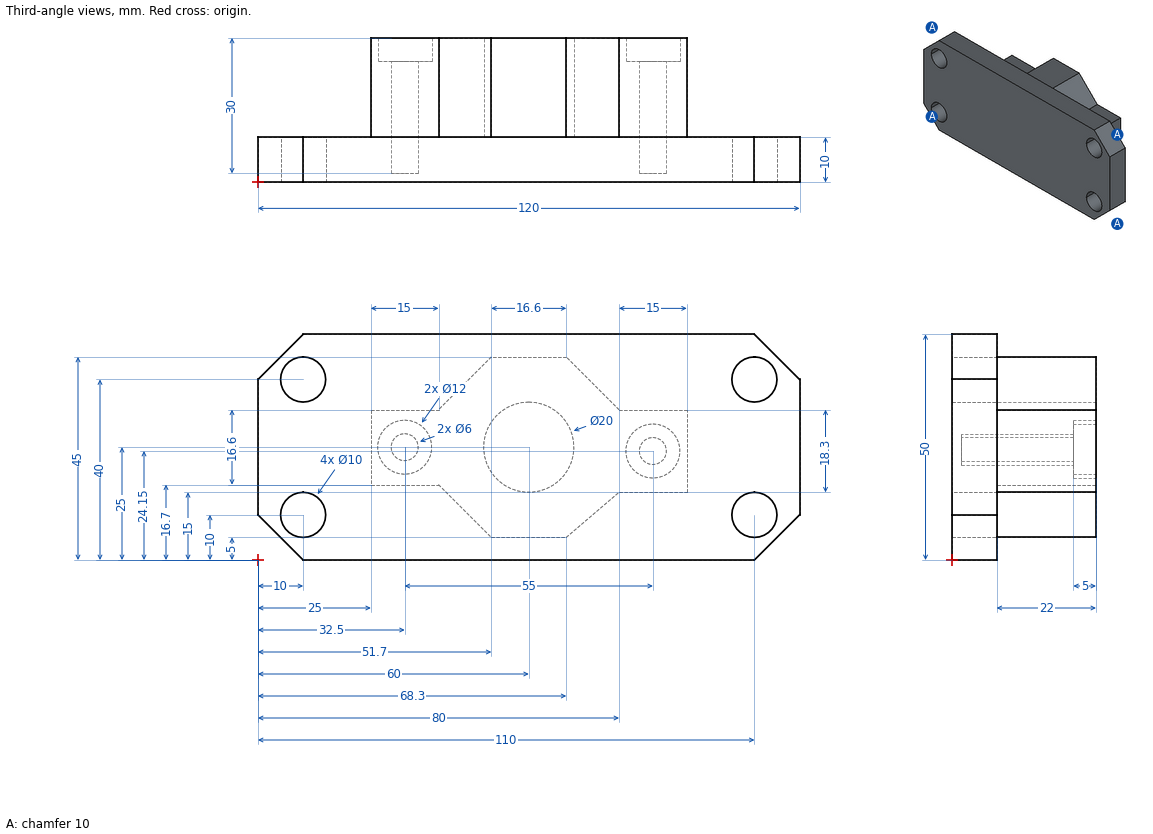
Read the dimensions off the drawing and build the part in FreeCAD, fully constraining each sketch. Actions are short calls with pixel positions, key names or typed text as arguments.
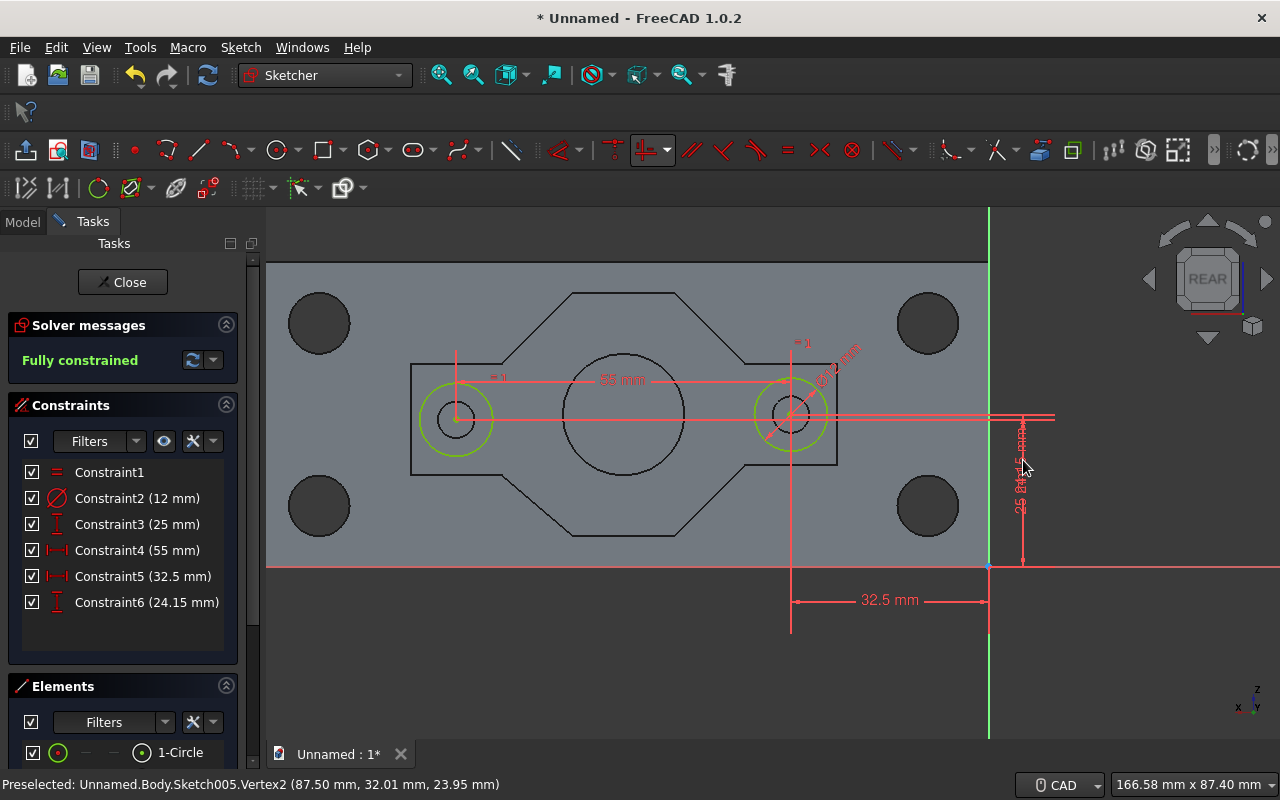
click(123, 282)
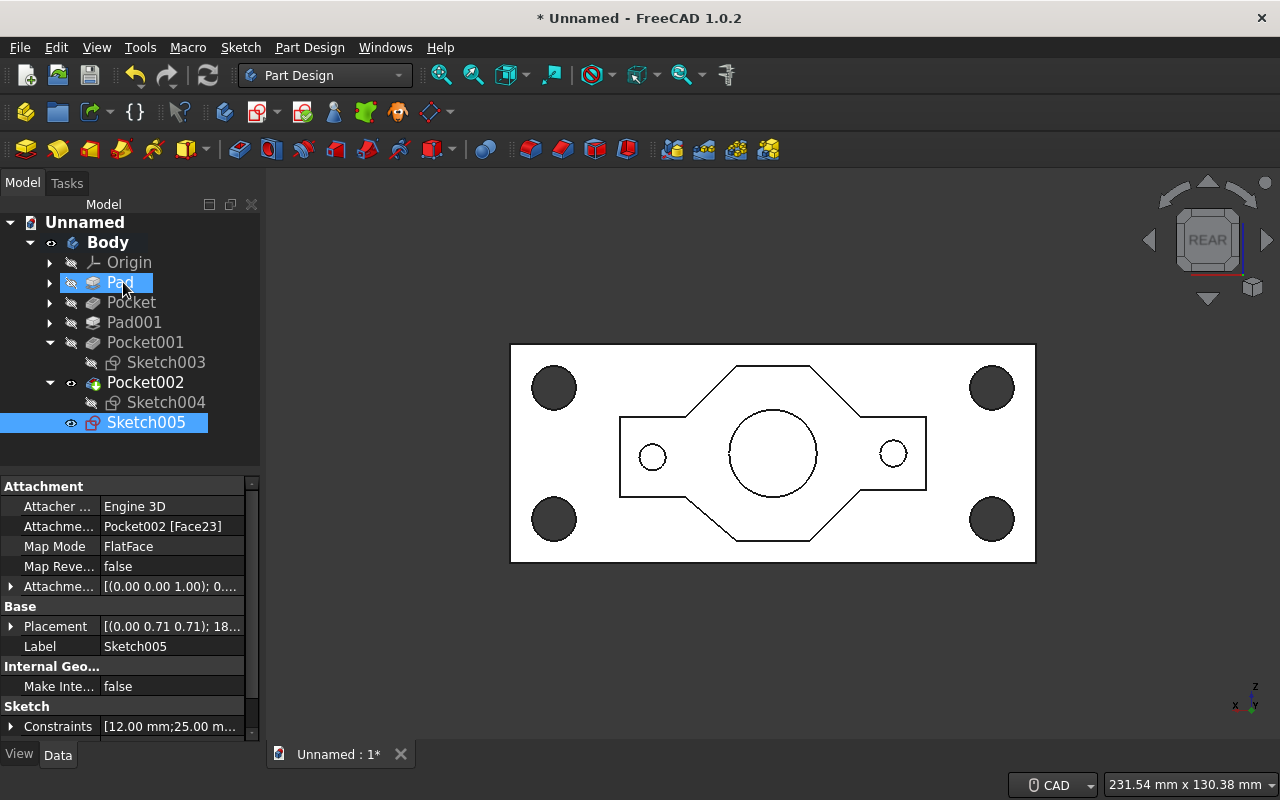
click(240, 150)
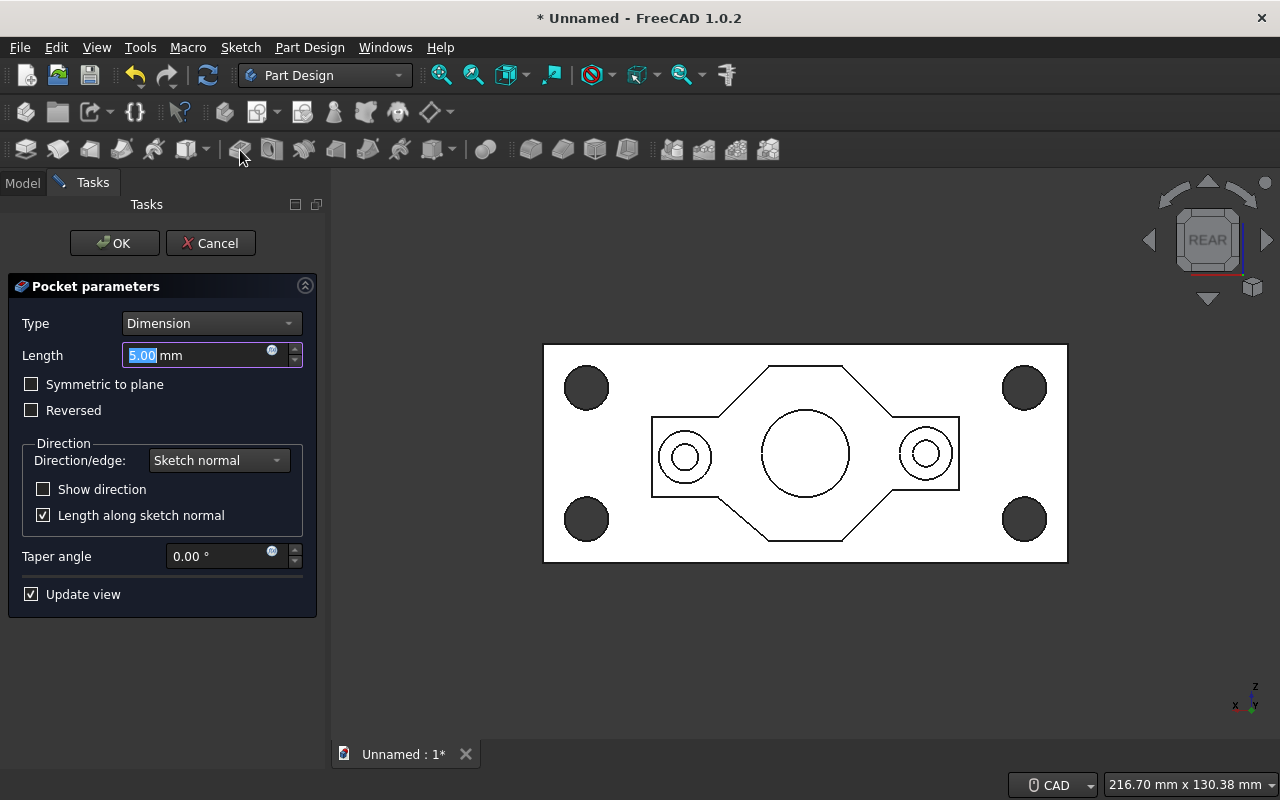
text(5)
key(Tab)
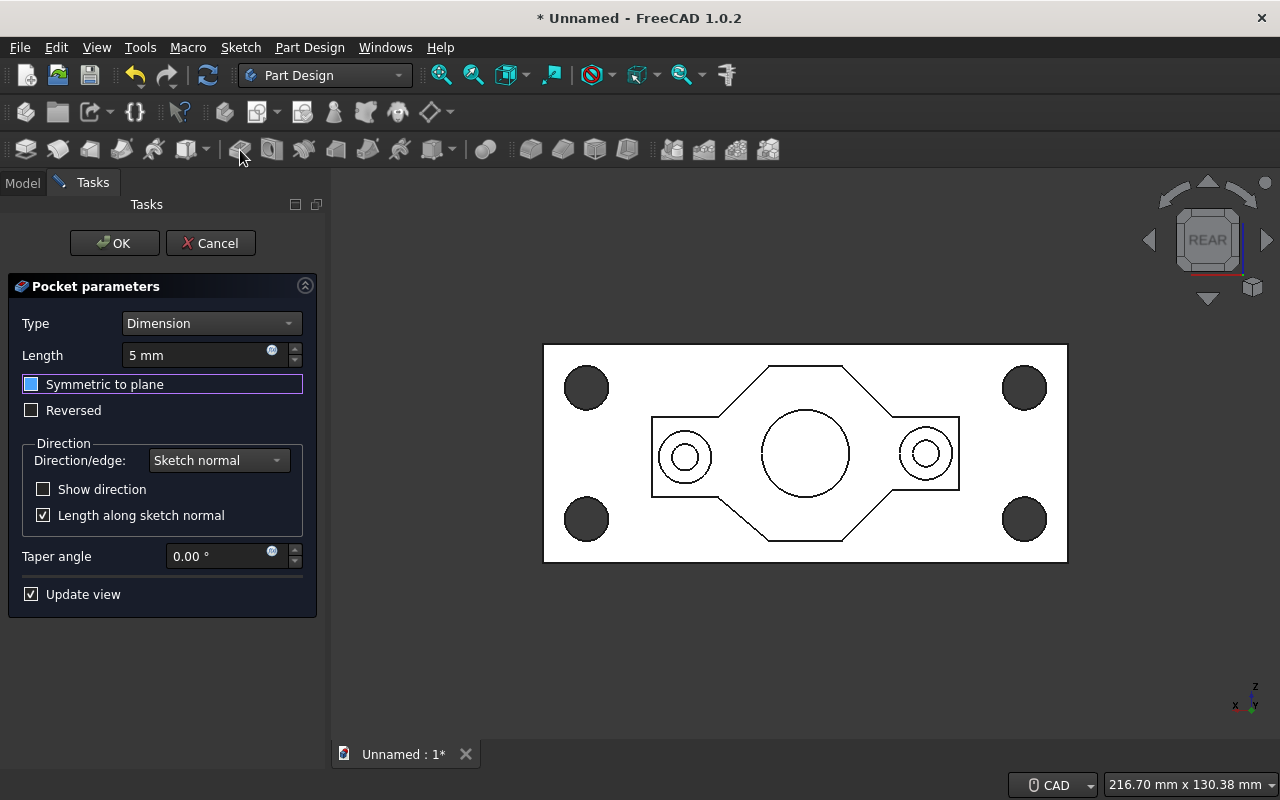
click(115, 243)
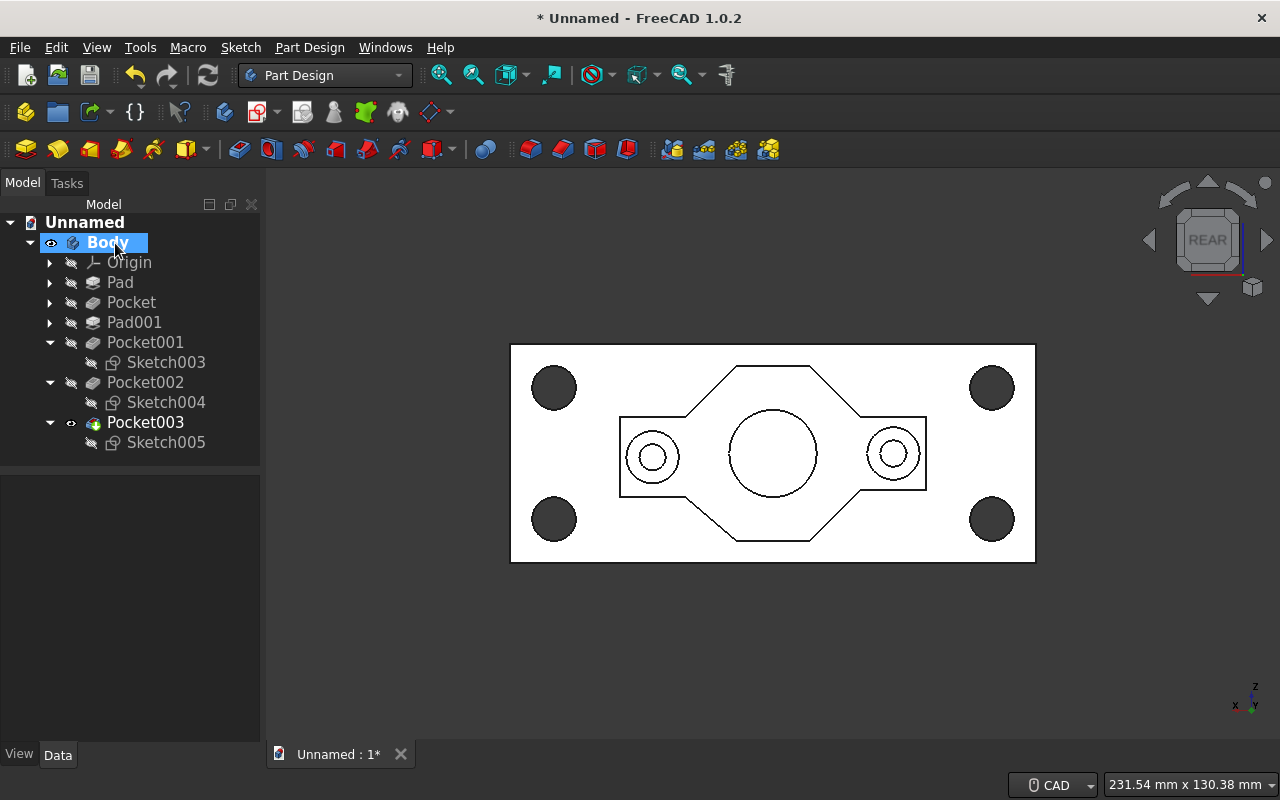
key(0)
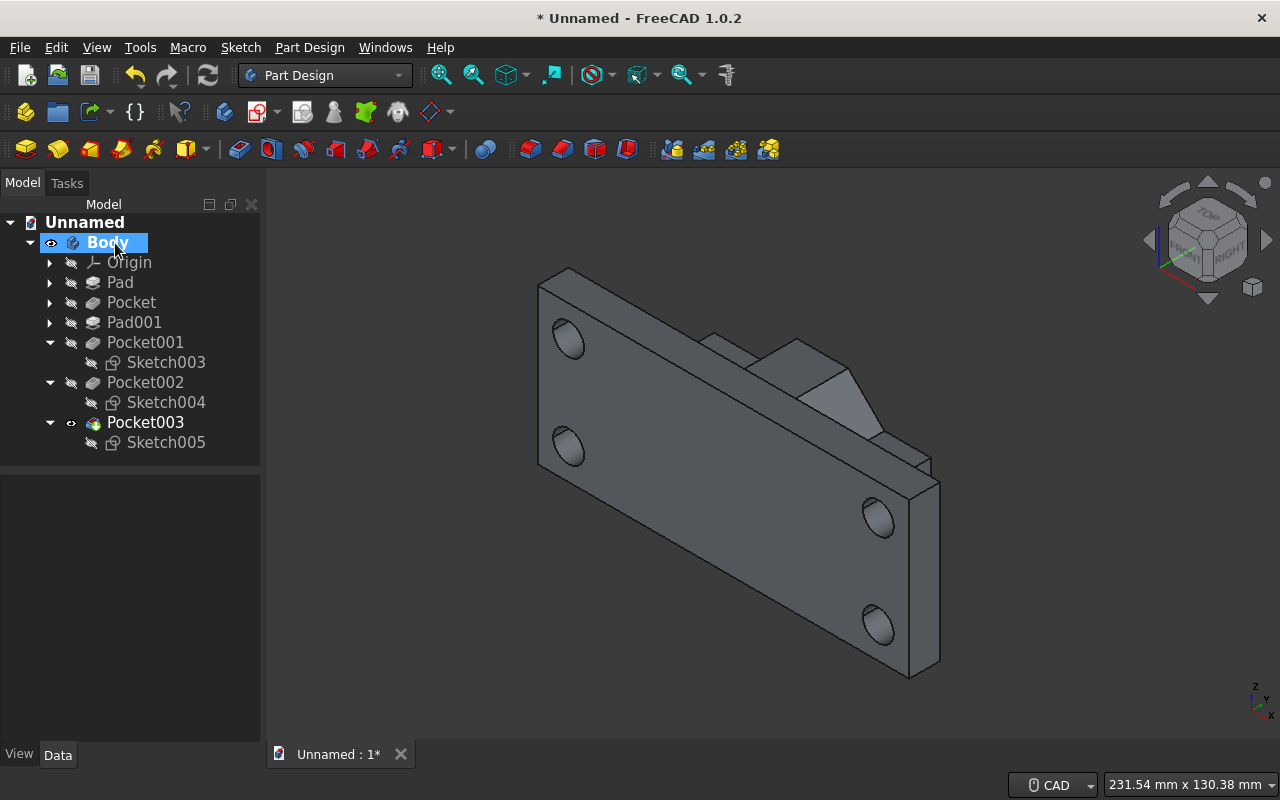
click(925, 490)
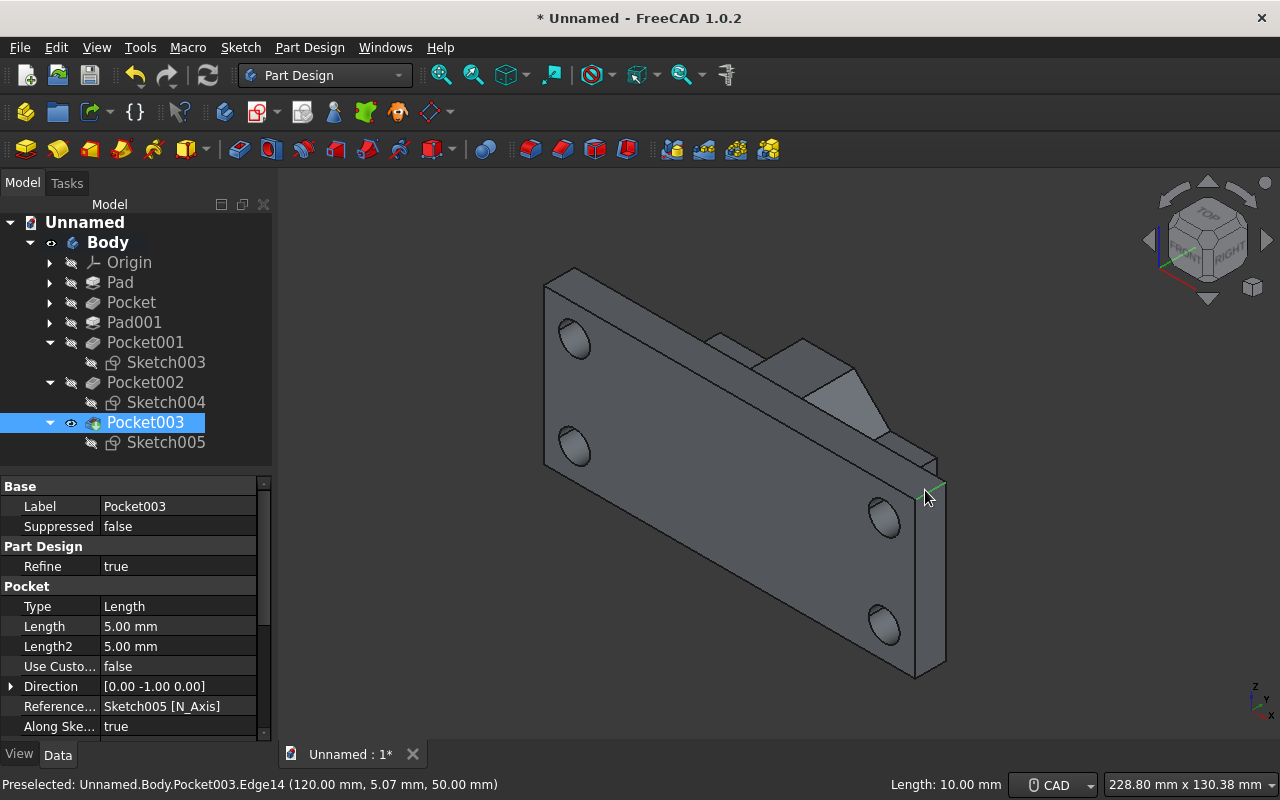
key(2)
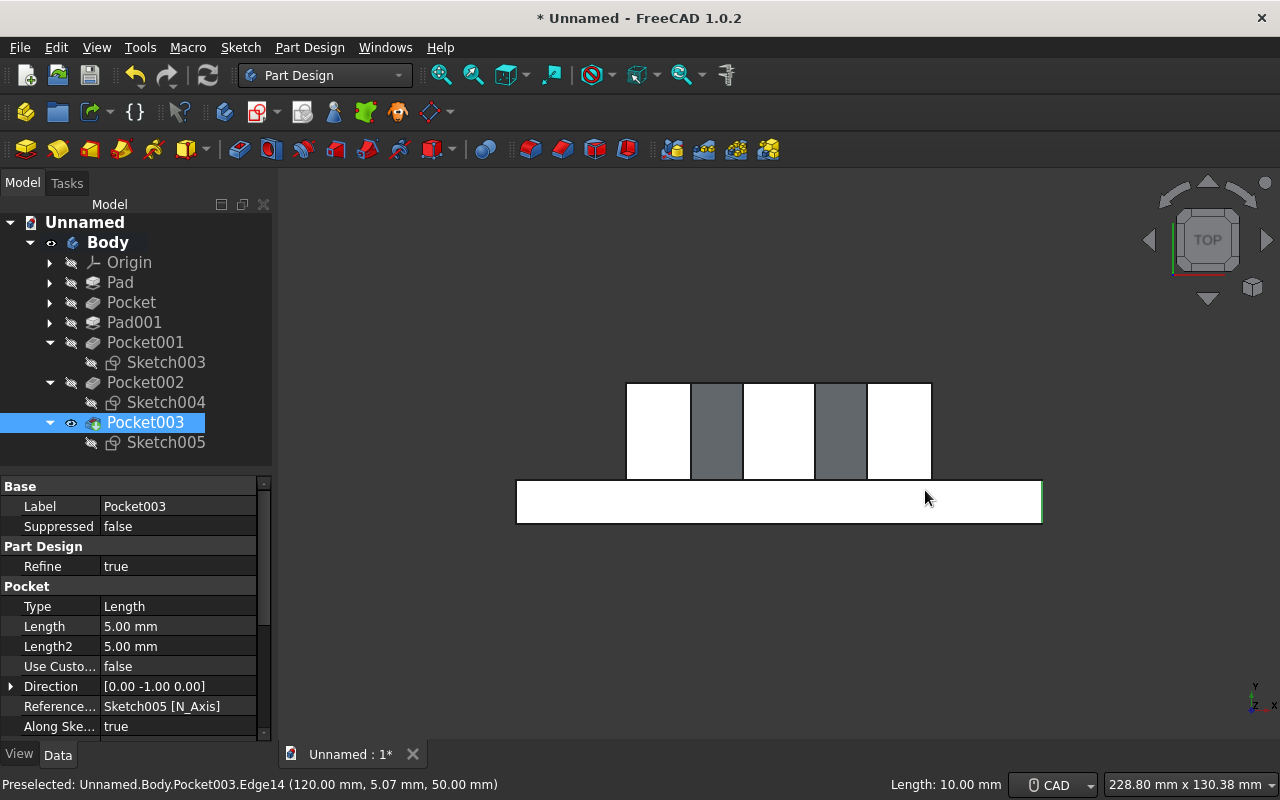
click(516, 501, ctrl)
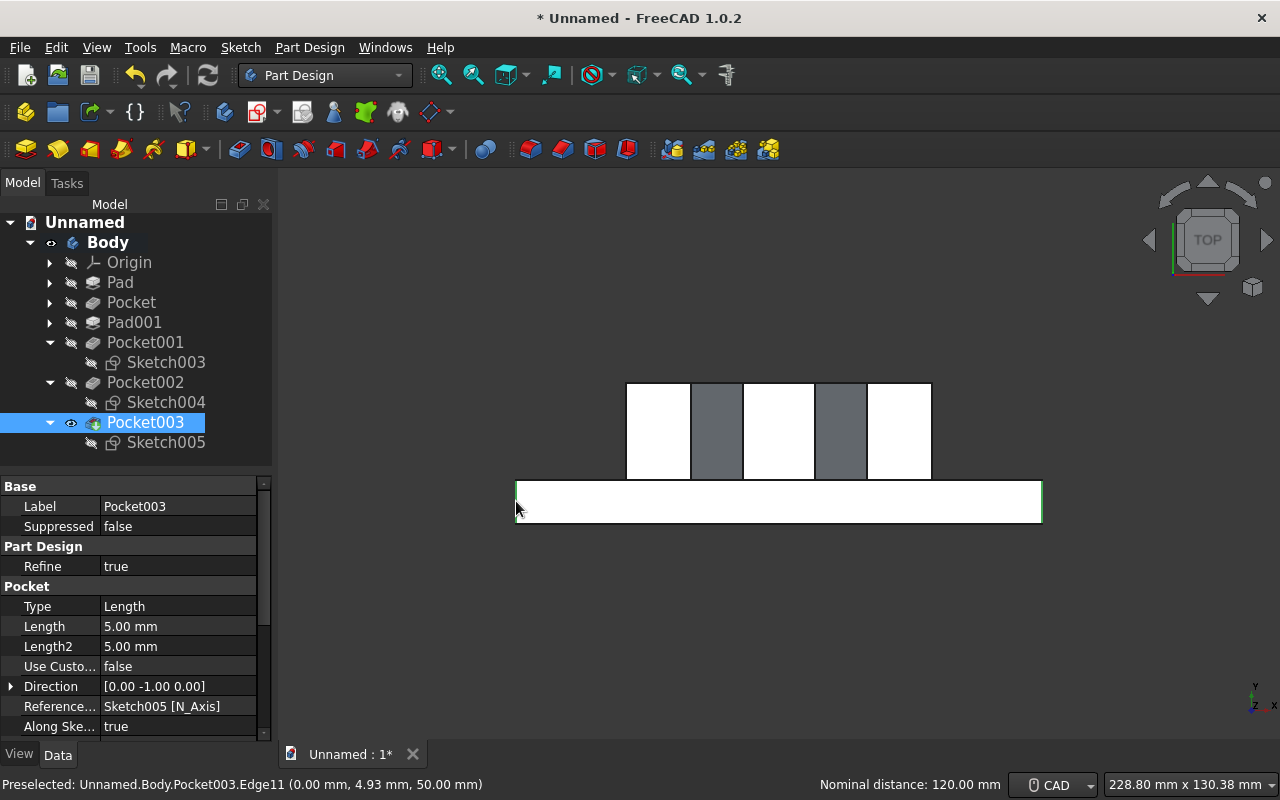
key(1)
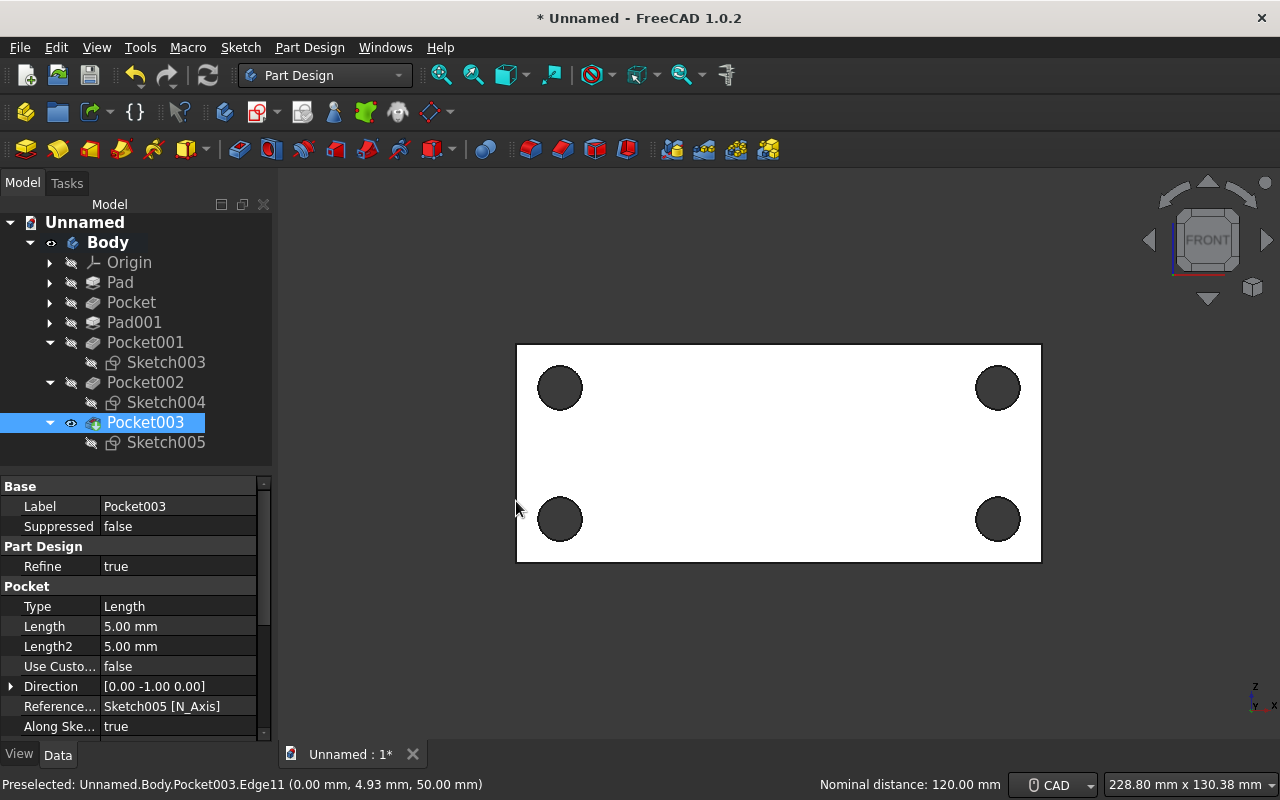
key(3)